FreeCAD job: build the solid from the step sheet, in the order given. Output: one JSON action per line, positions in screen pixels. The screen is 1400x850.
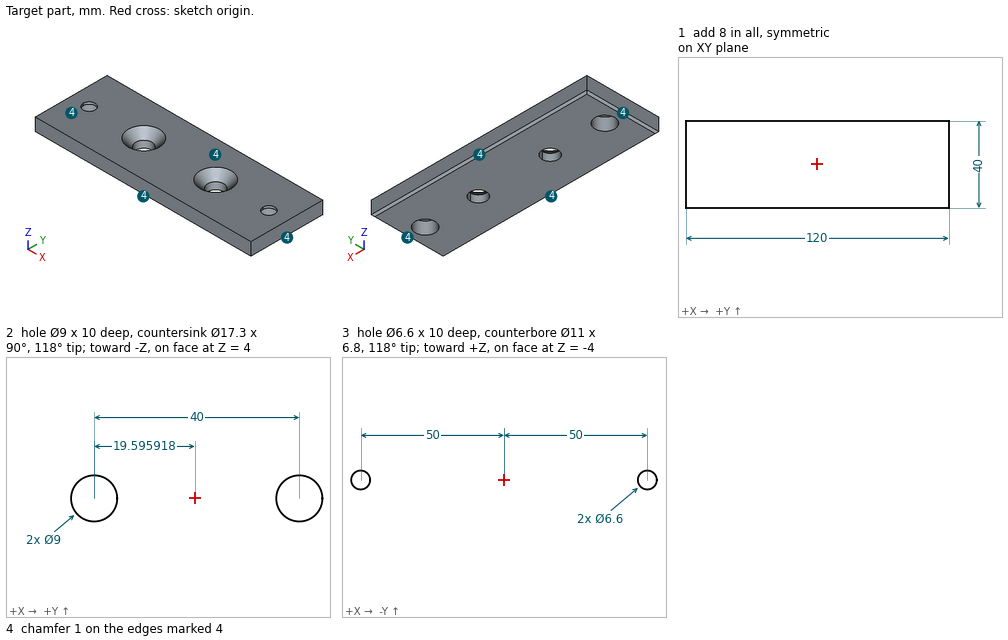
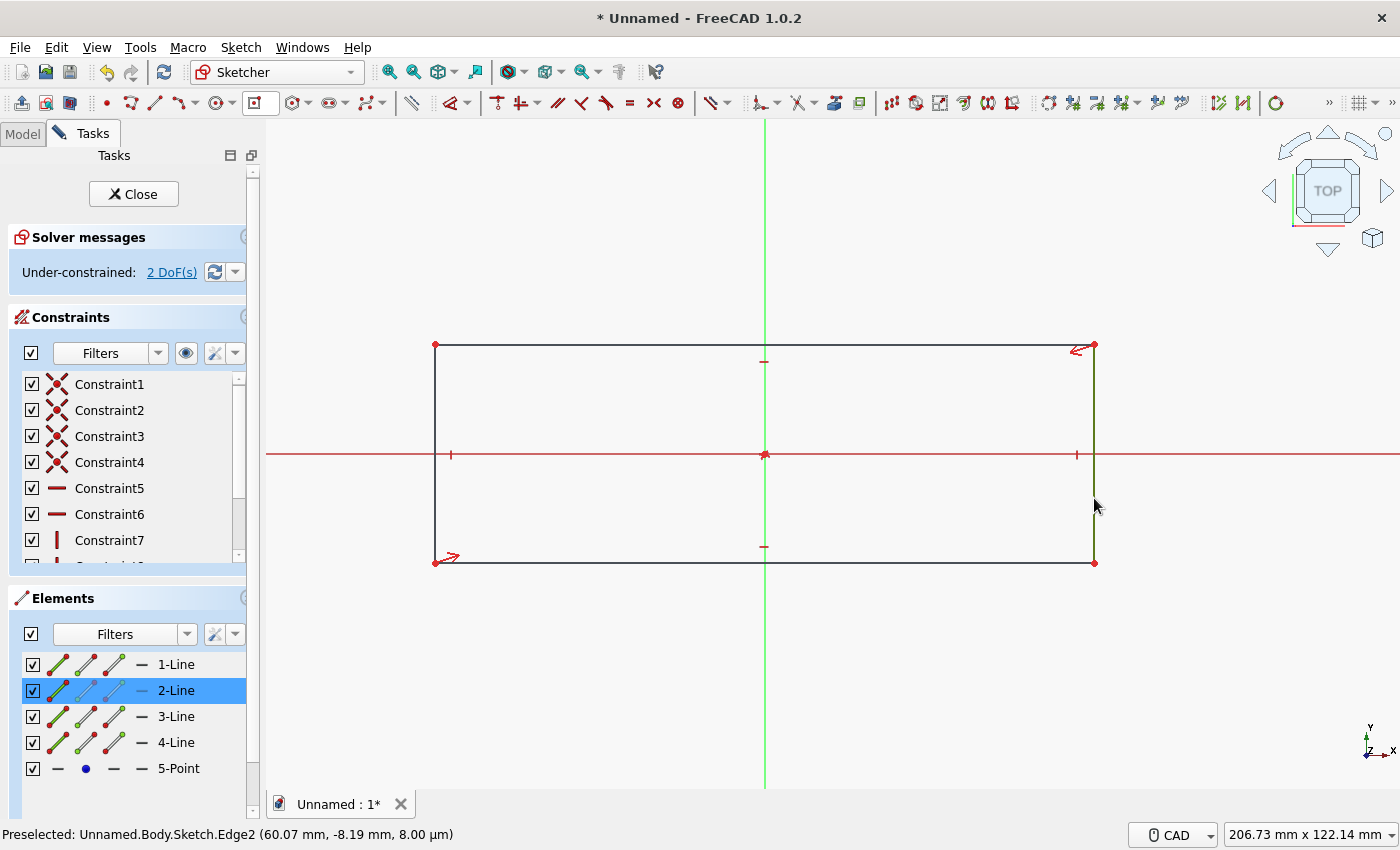
{"action": "key", "text": "i"}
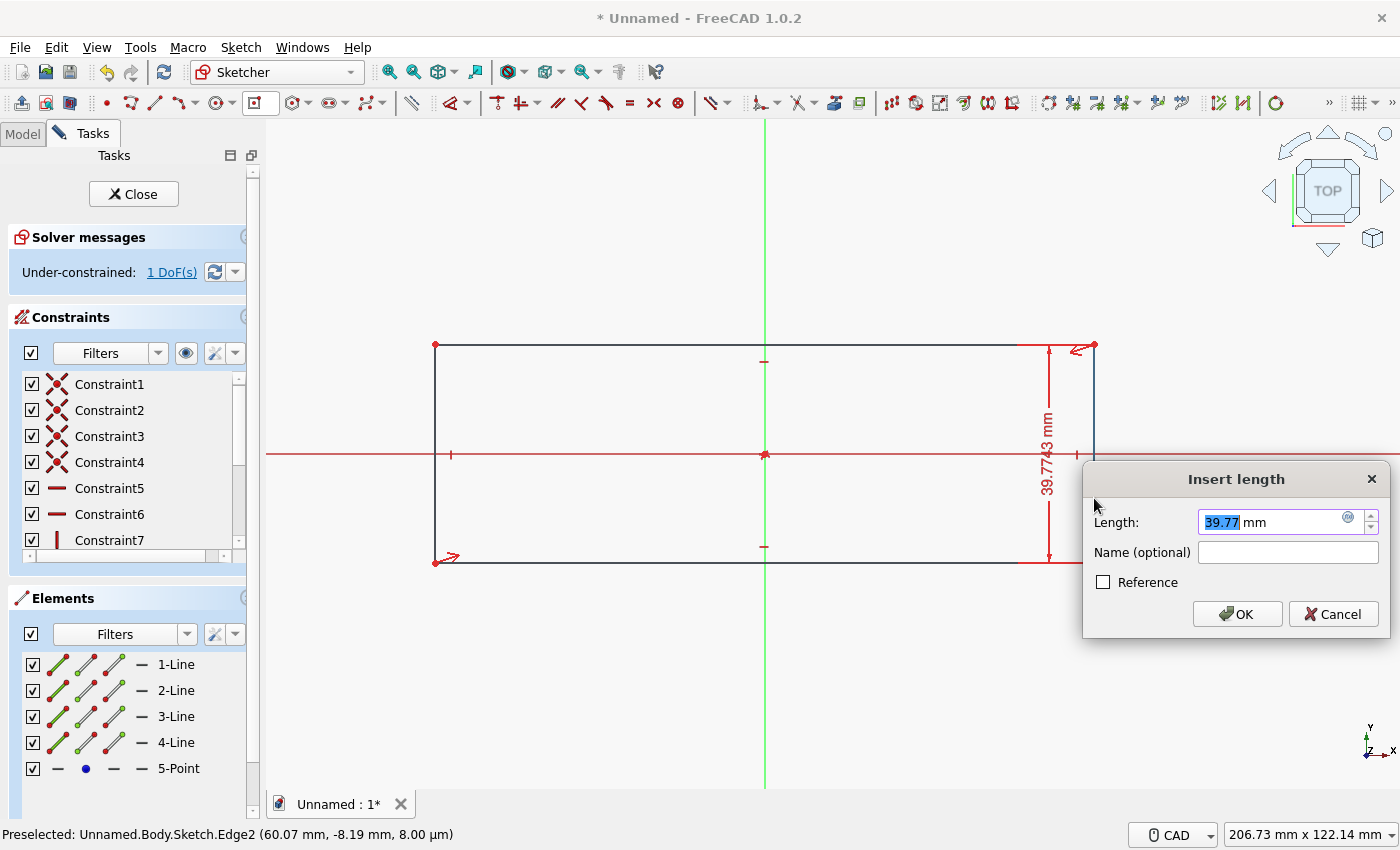
{"action": "type", "text": "40"}
{"action": "key", "text": "Return"}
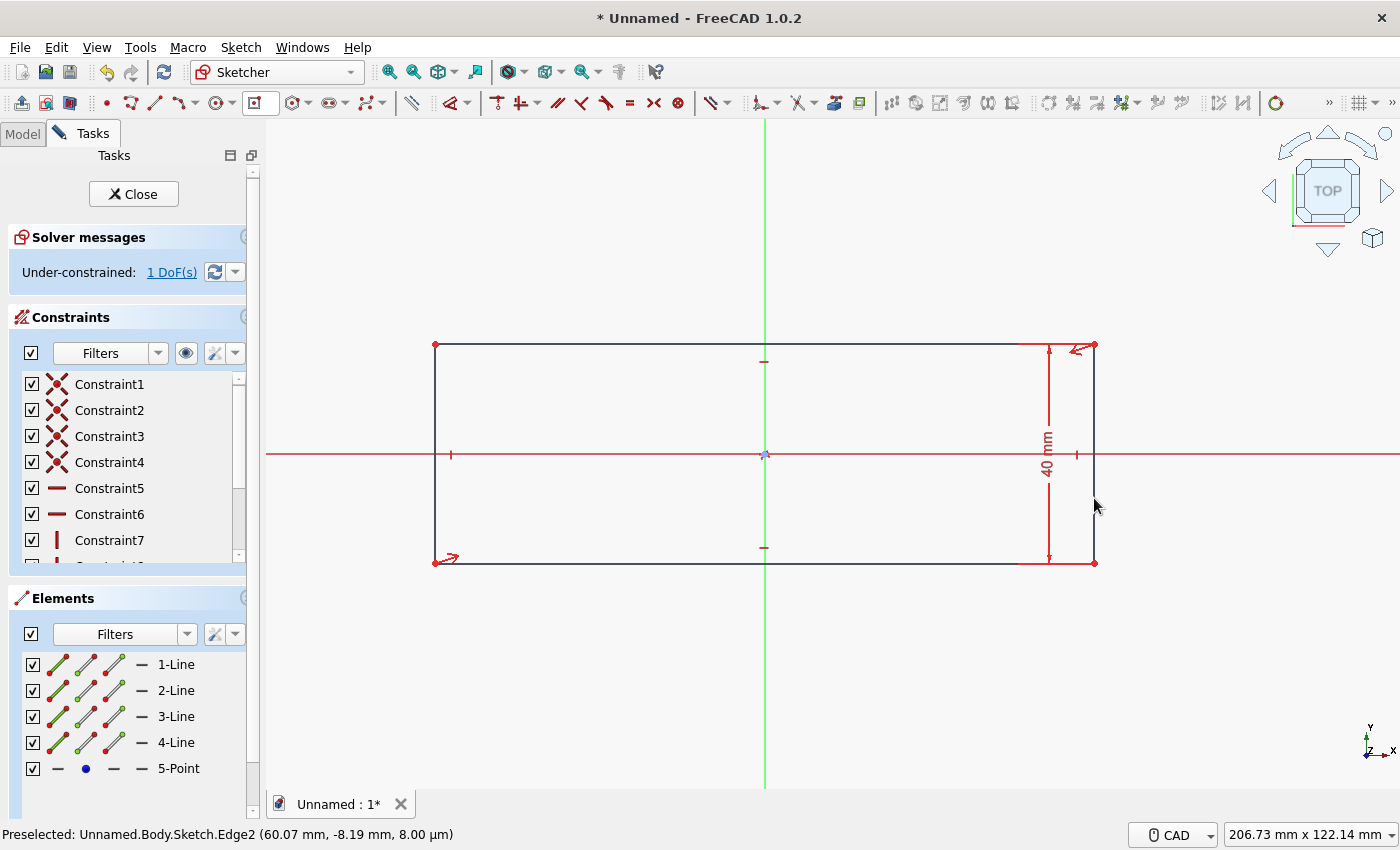
{"action": "left_click", "coordinate": [633, 564]}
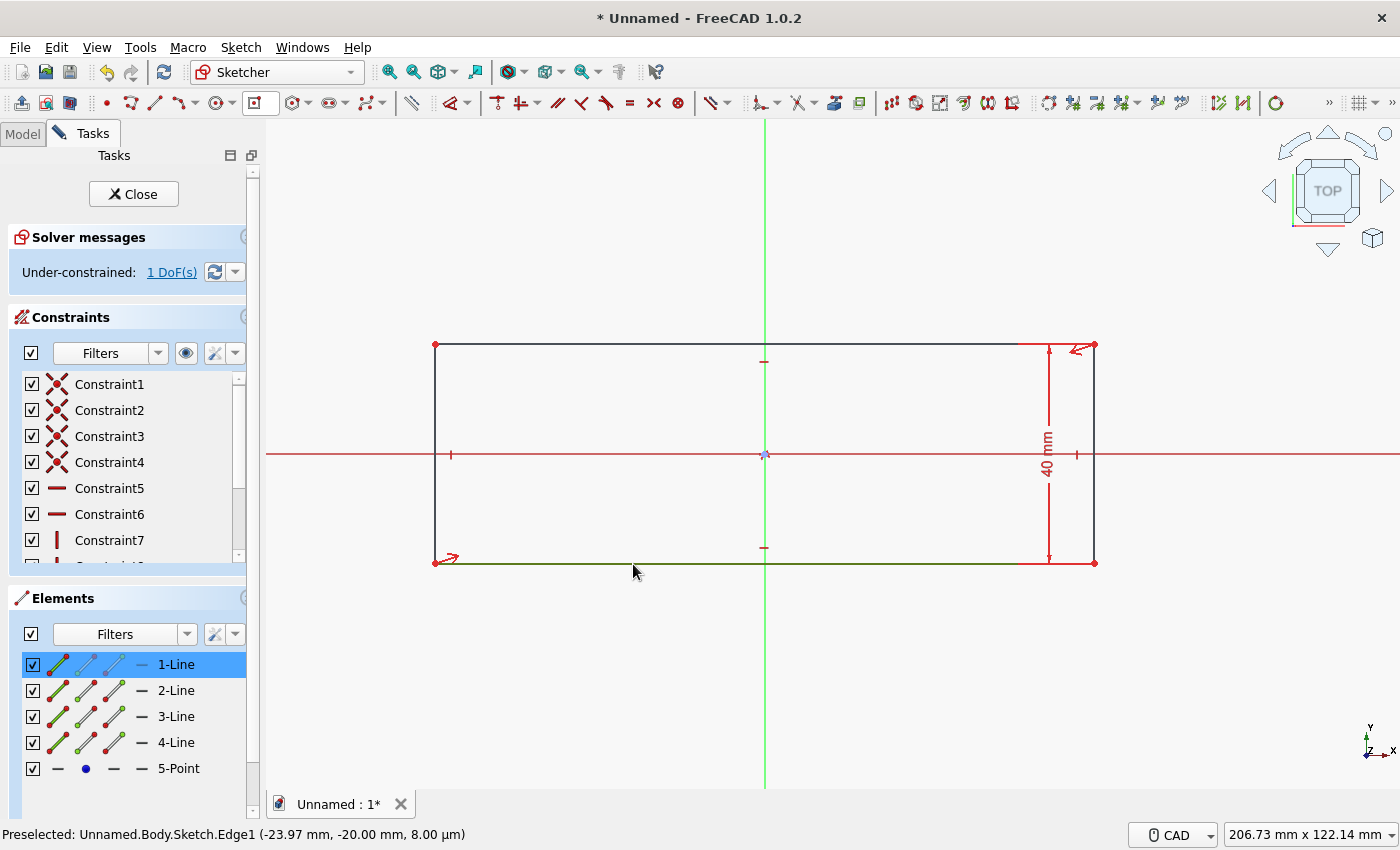
{"action": "key", "text": "l"}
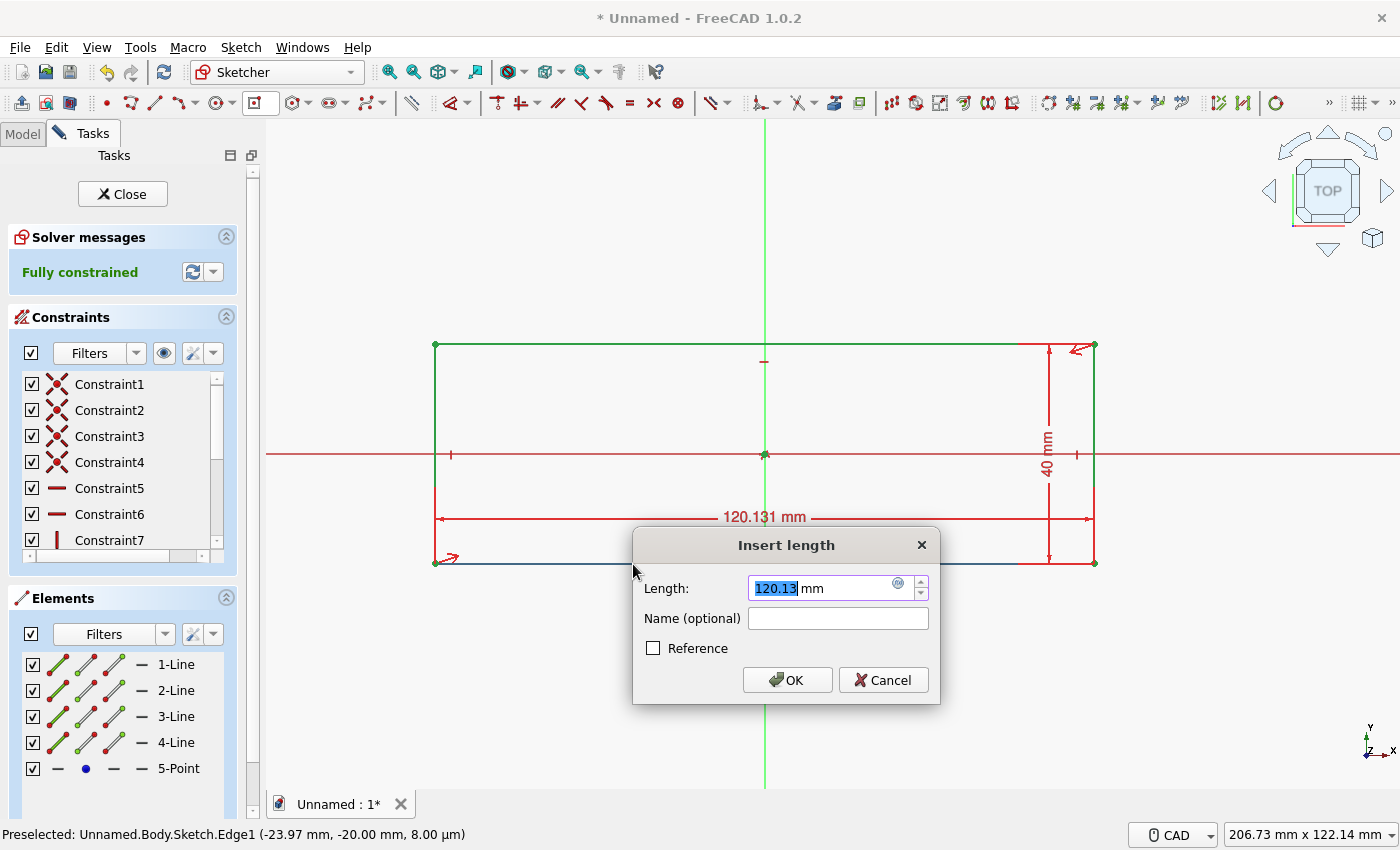
{"action": "type", "text": "120"}
{"action": "key", "text": "Return"}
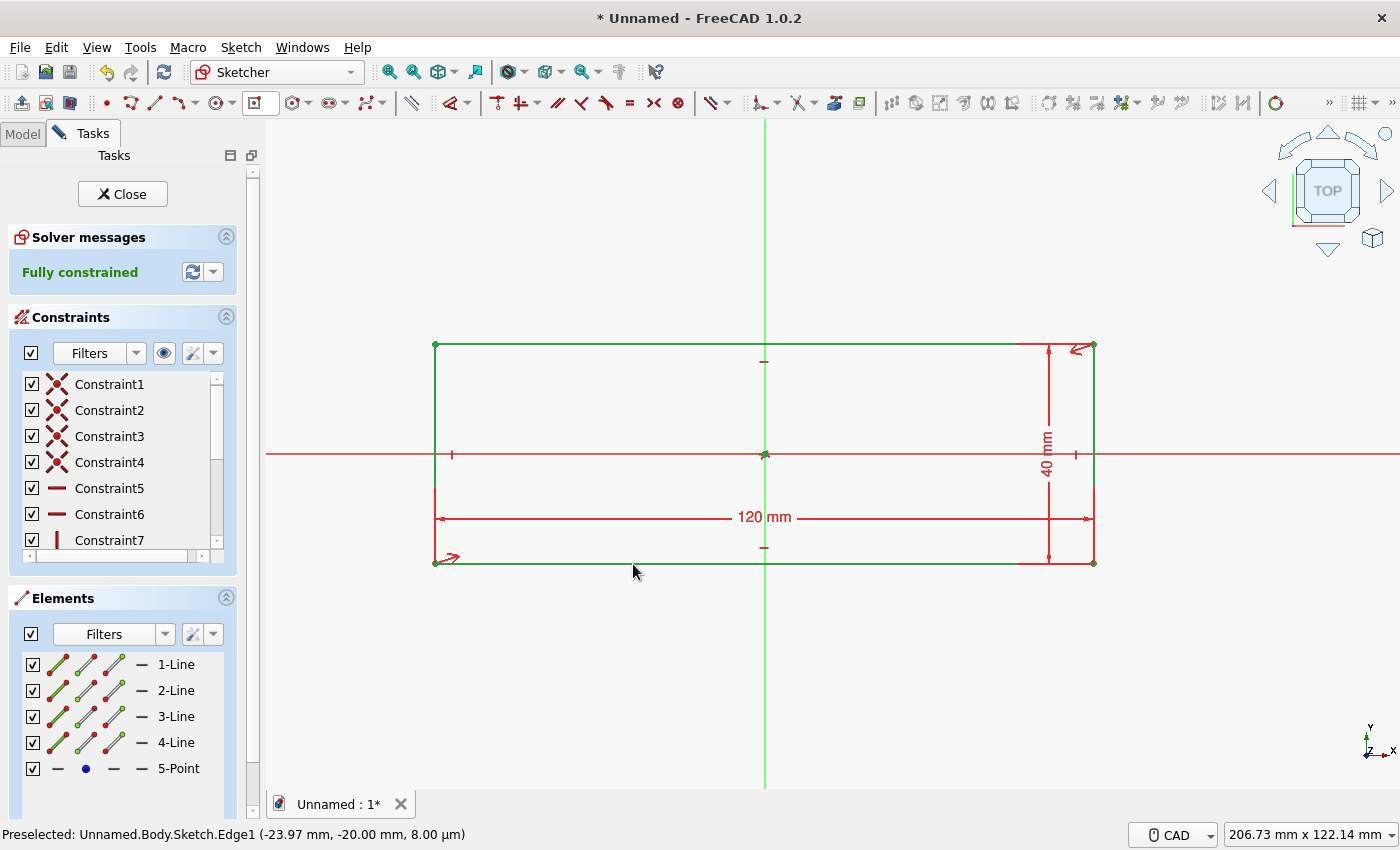
{"action": "left_click", "coordinate": [123, 194]}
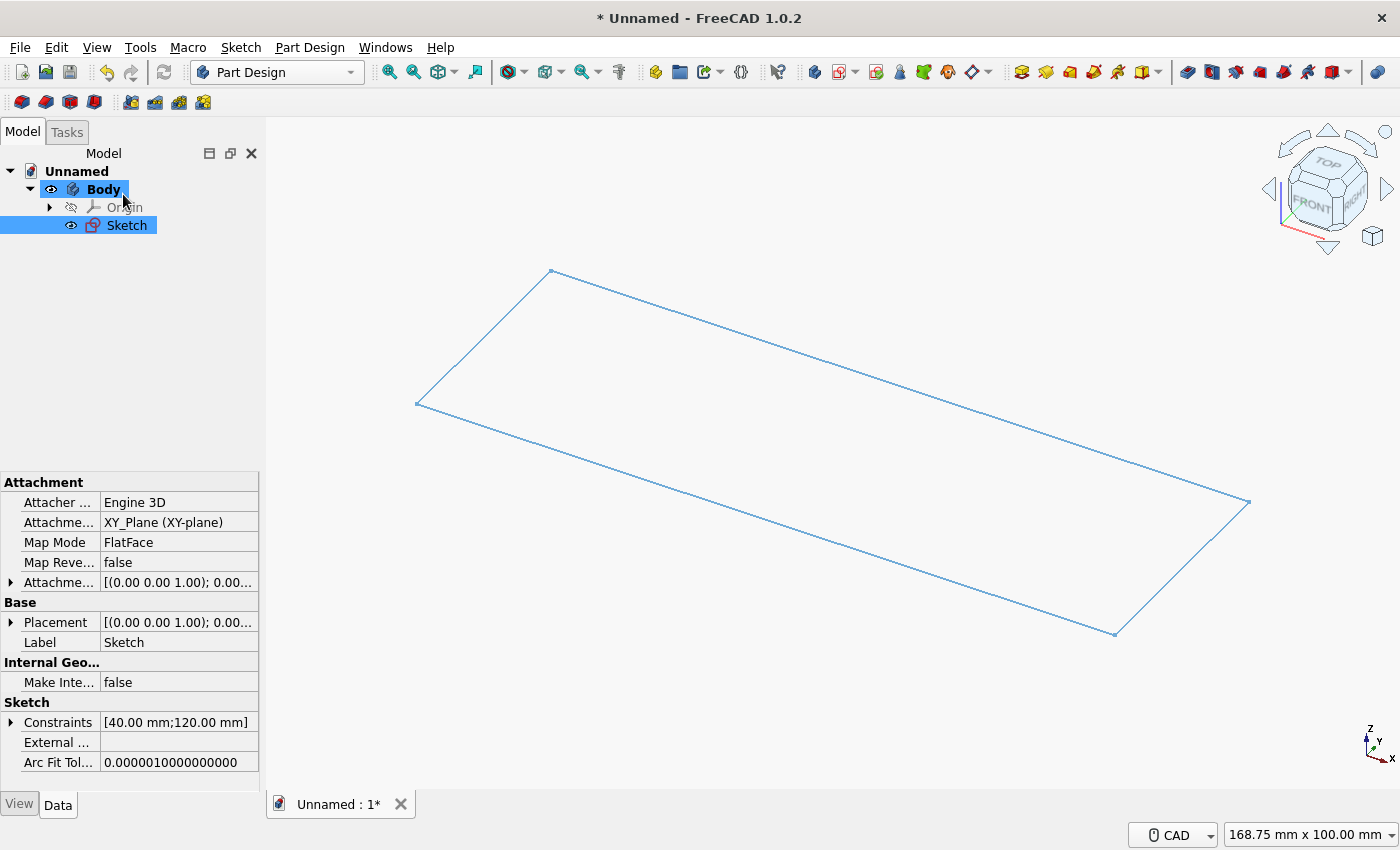
{"action": "left_click", "coordinate": [1022, 72]}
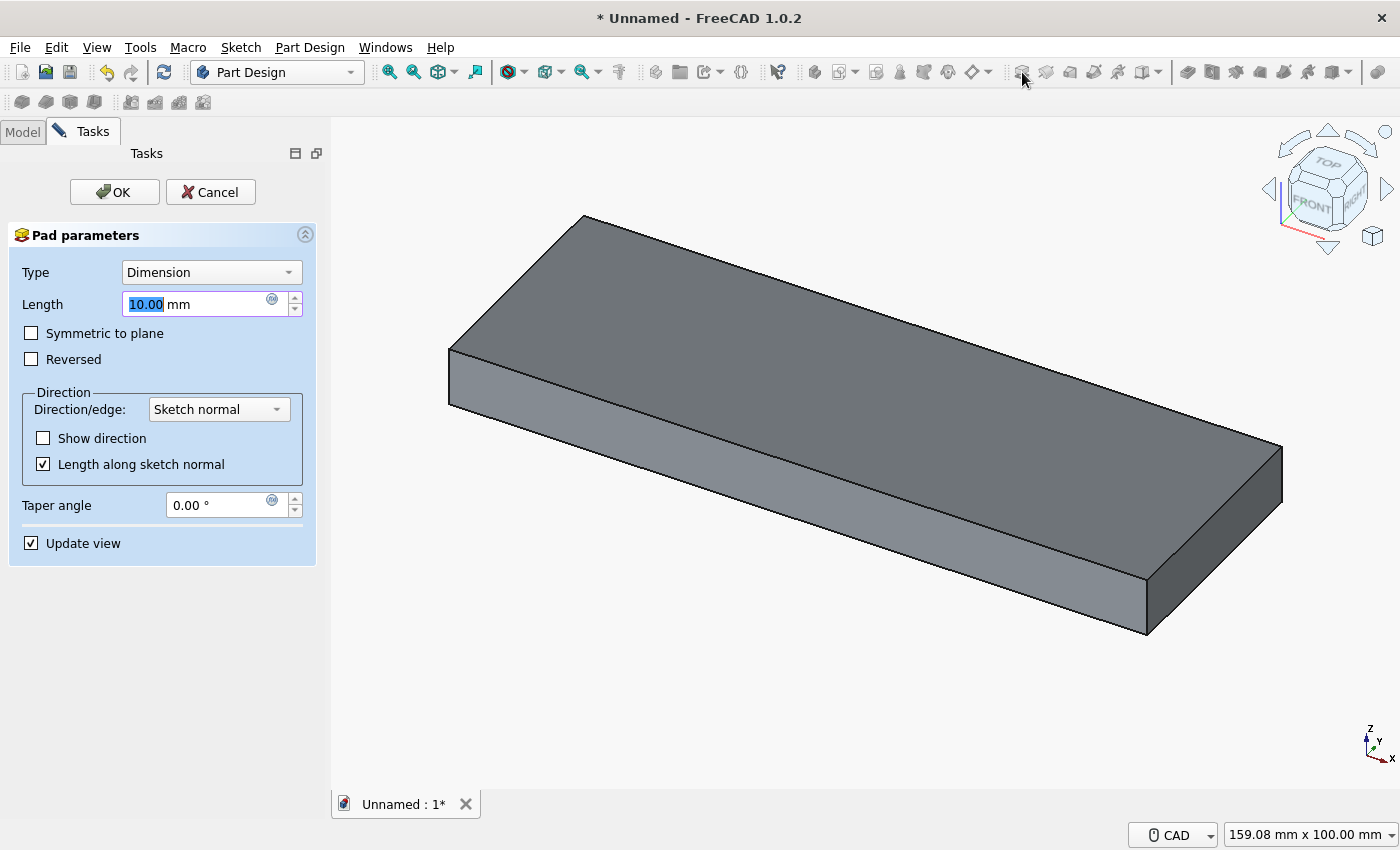
{"action": "type", "text": "8"}
{"action": "key", "text": "Tab"}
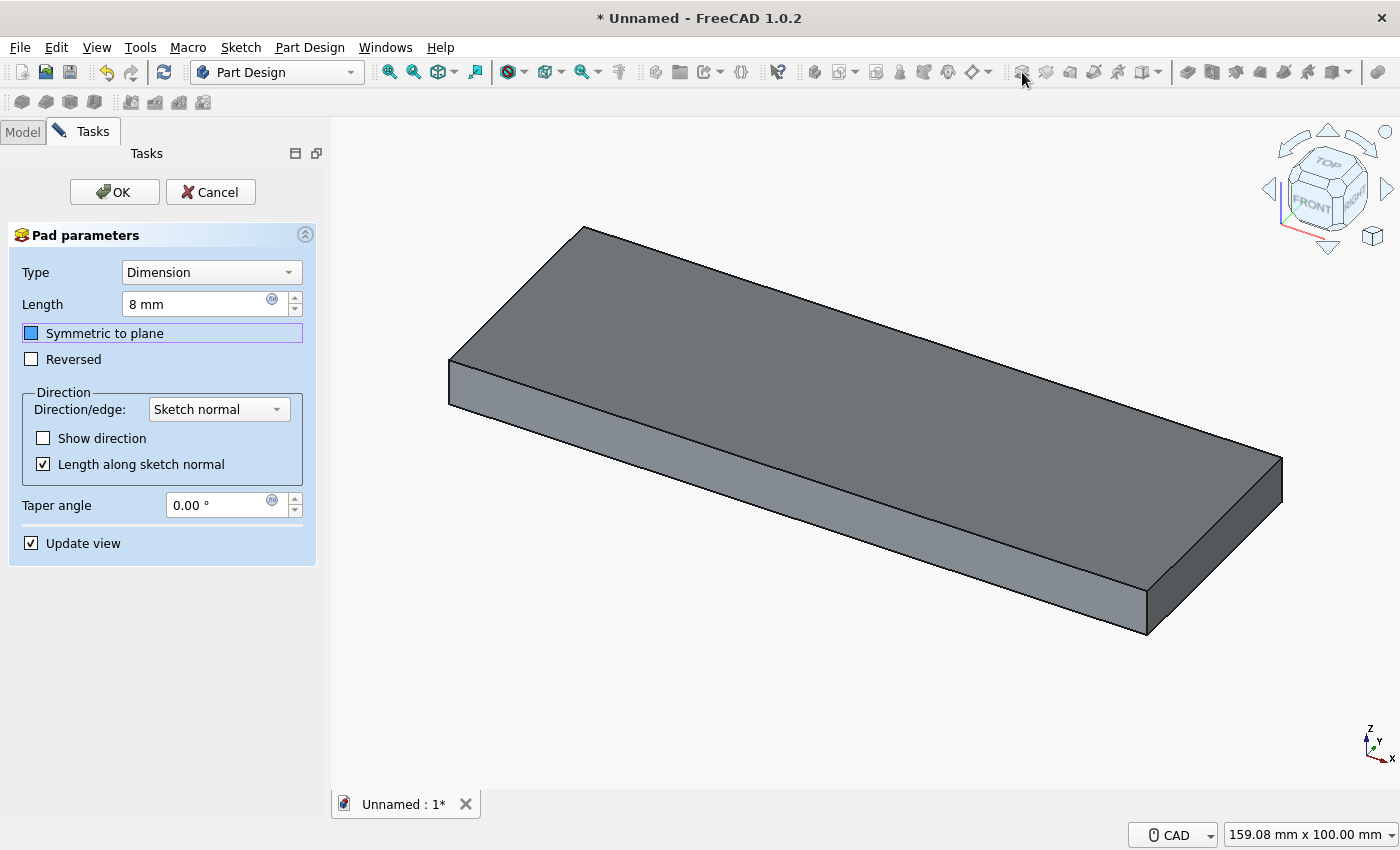
{"action": "left_click", "coordinate": [30, 333]}